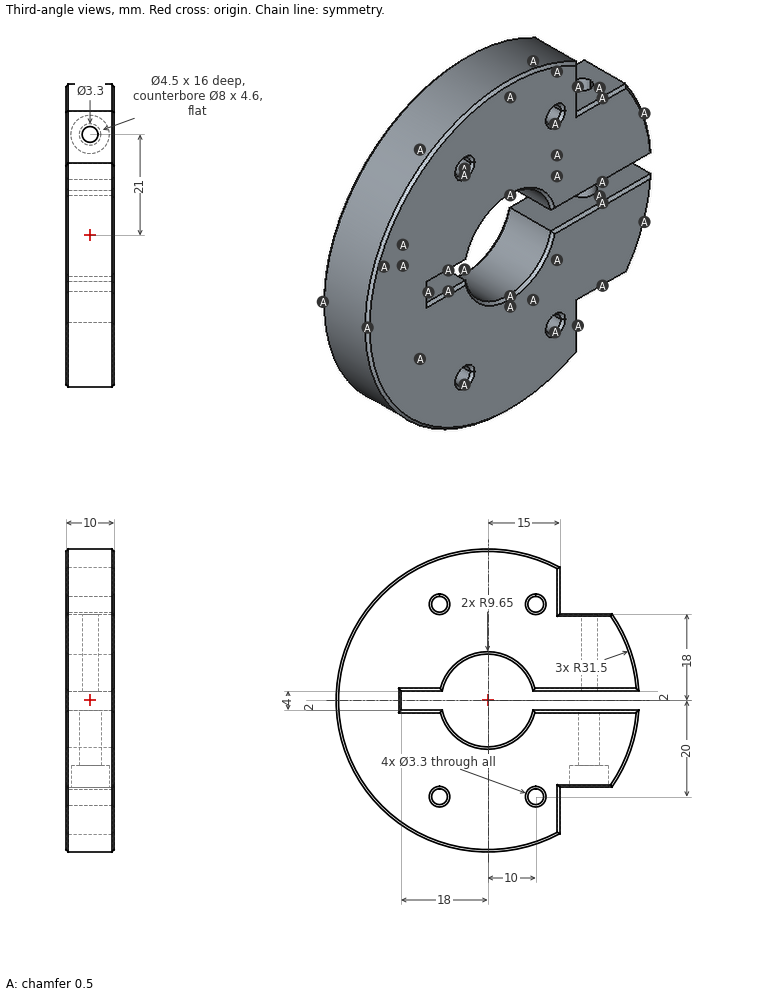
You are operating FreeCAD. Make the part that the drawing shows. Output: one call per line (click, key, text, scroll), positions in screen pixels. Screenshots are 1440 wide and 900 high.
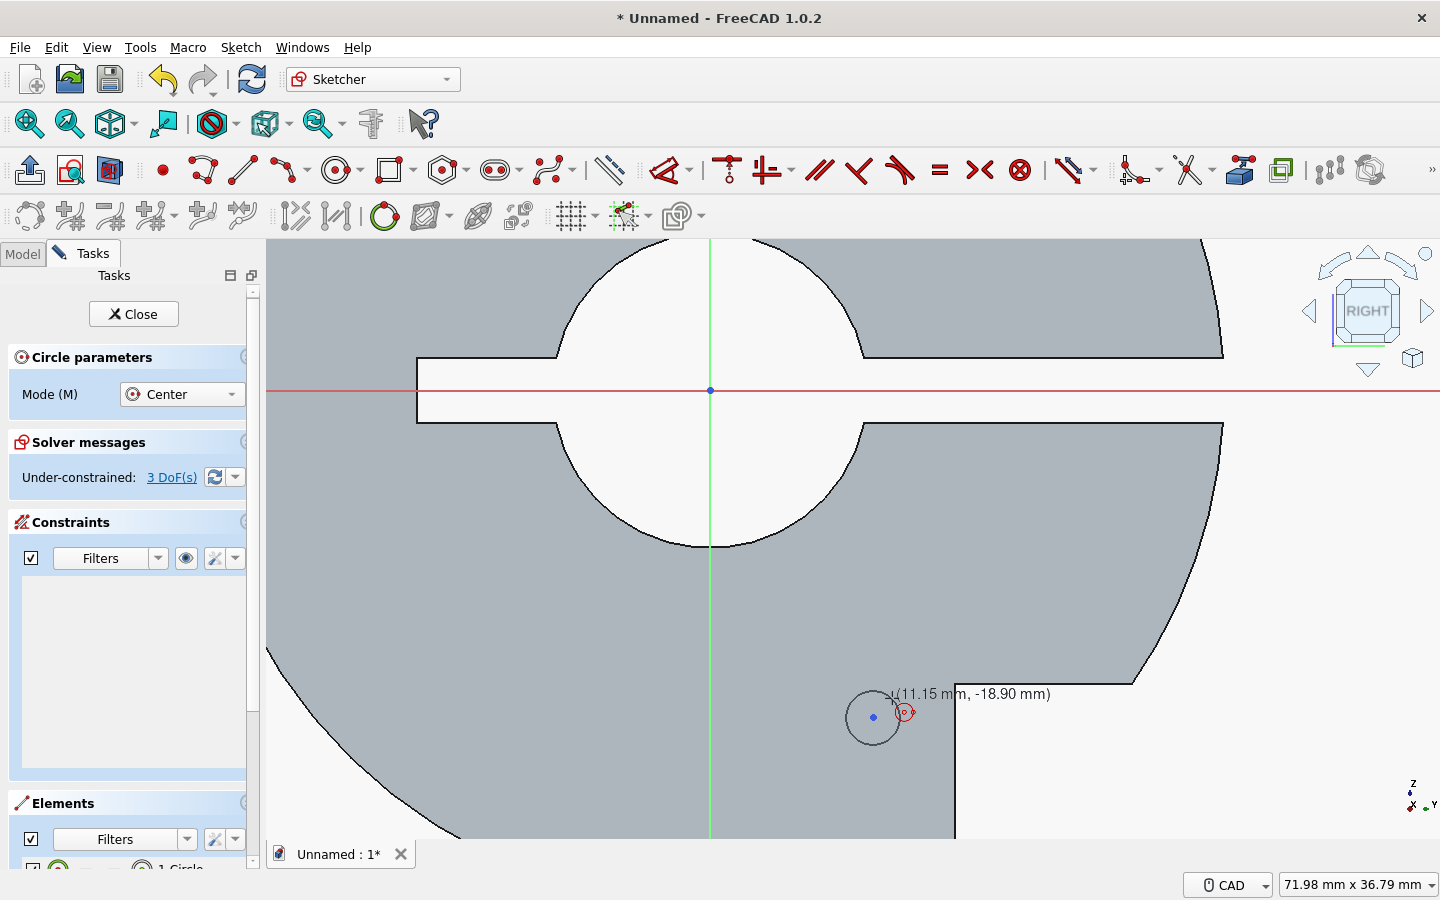
click(547, 717)
click(566, 698)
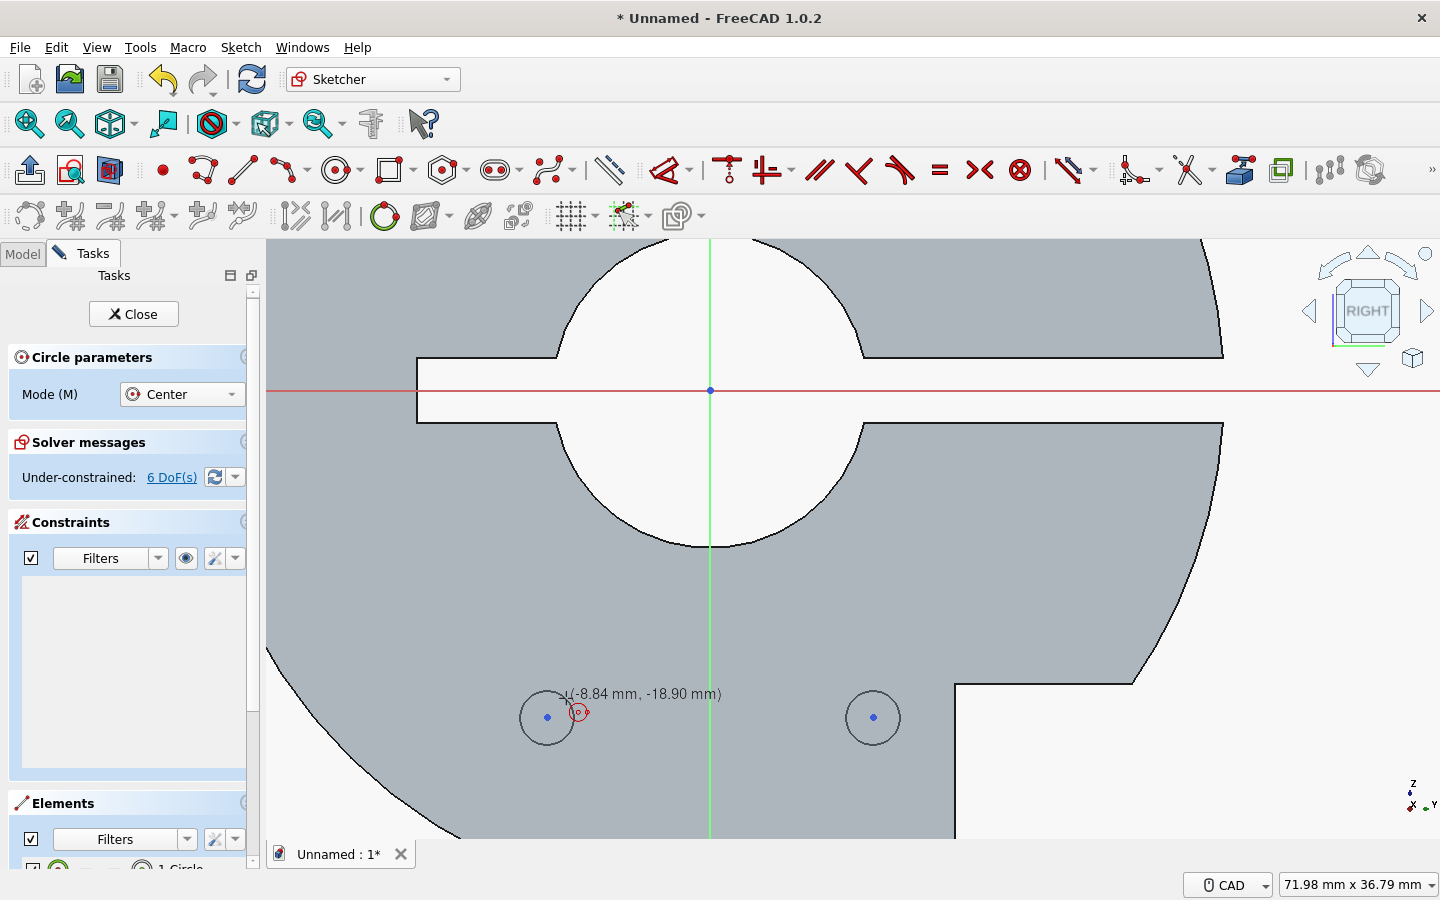
scroll(875, 719, down, 3)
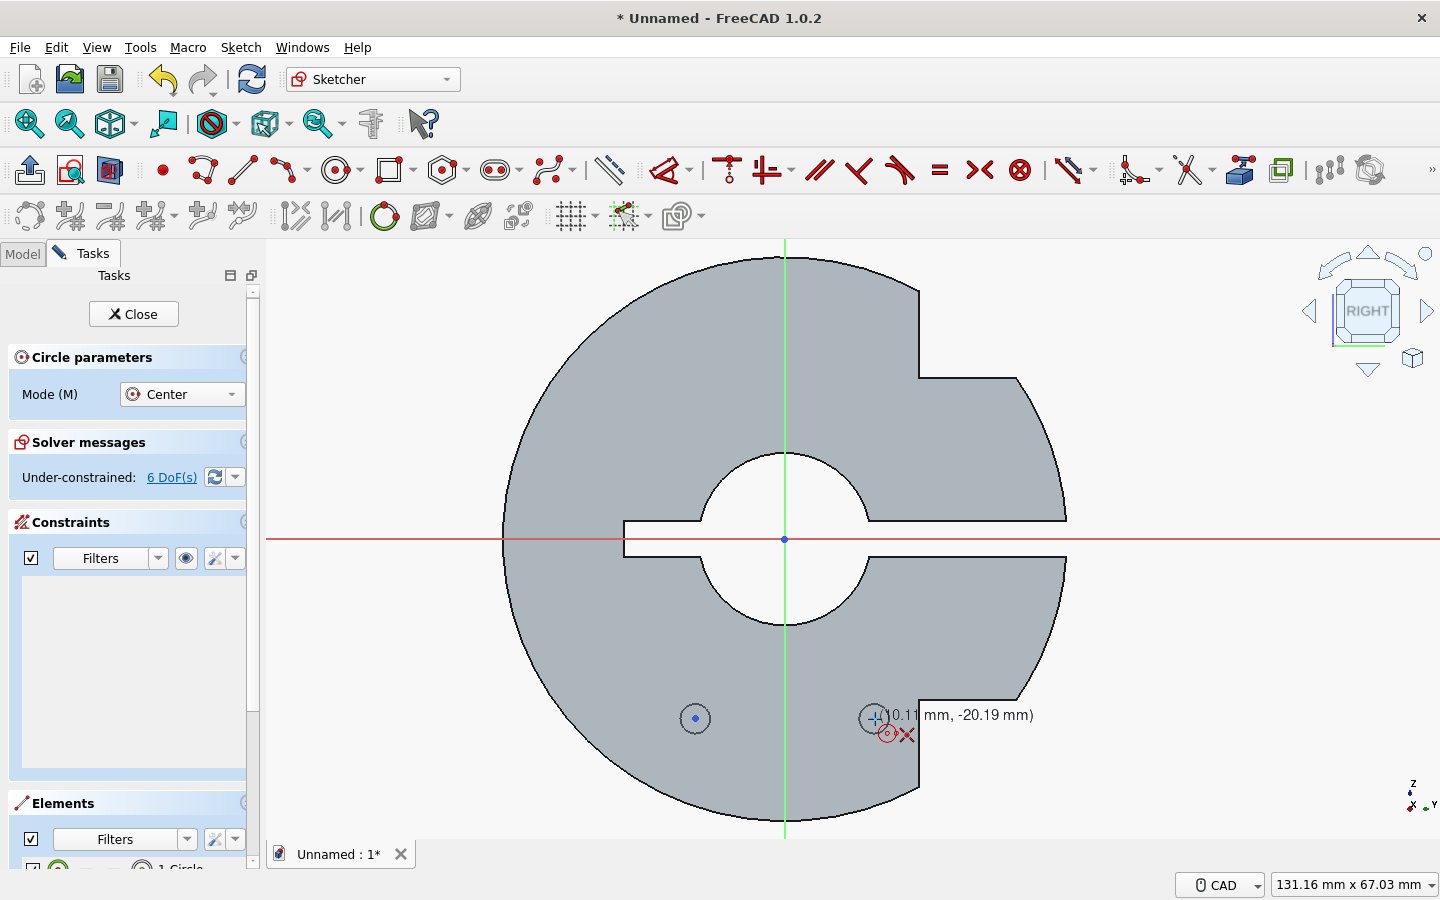
scroll(695, 360, up, 3)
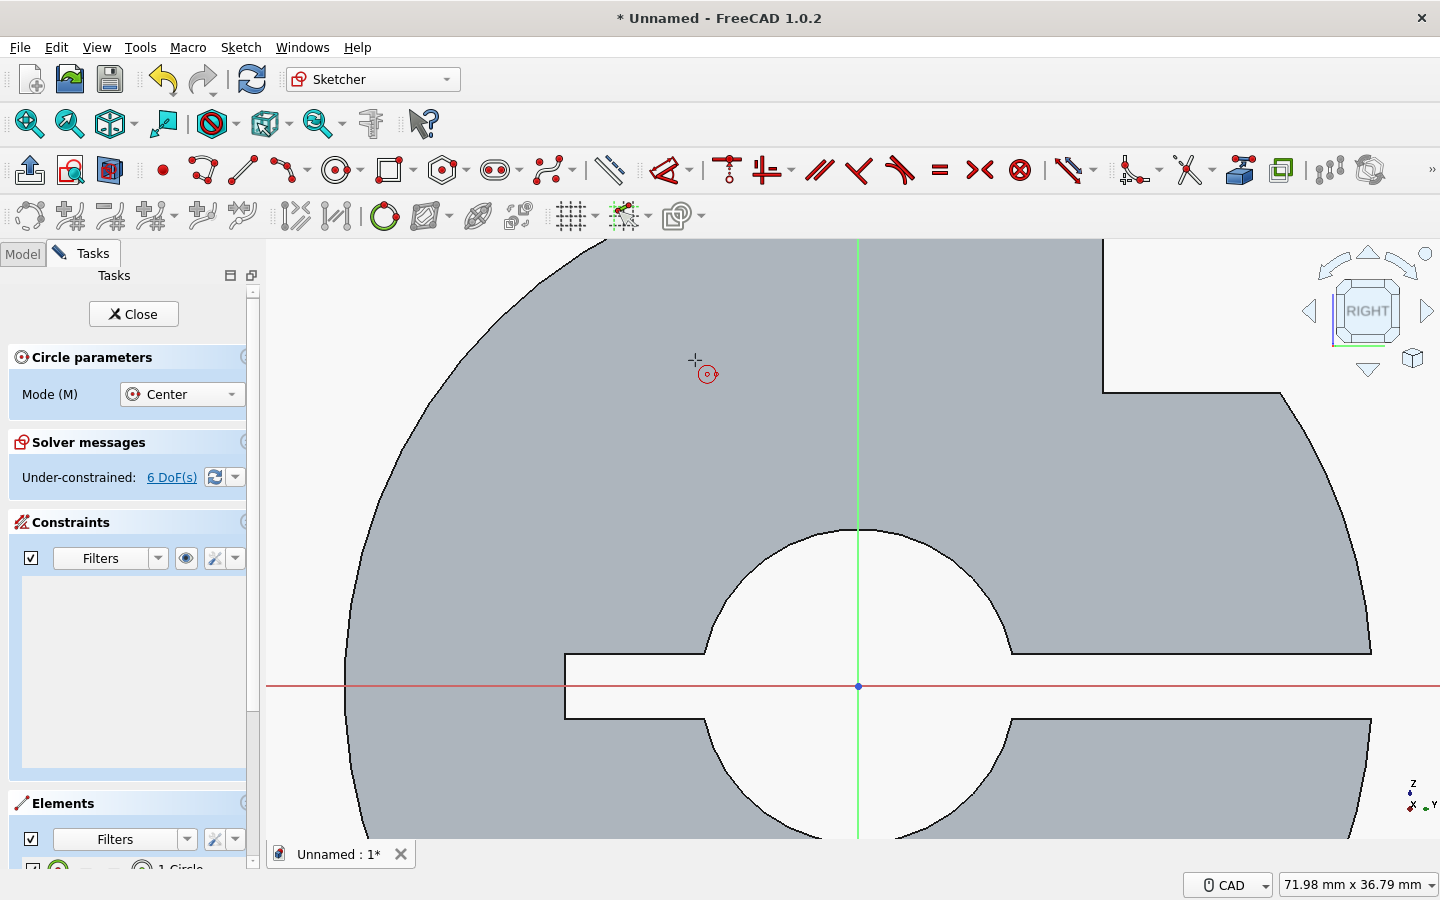
click(695, 360)
click(714, 341)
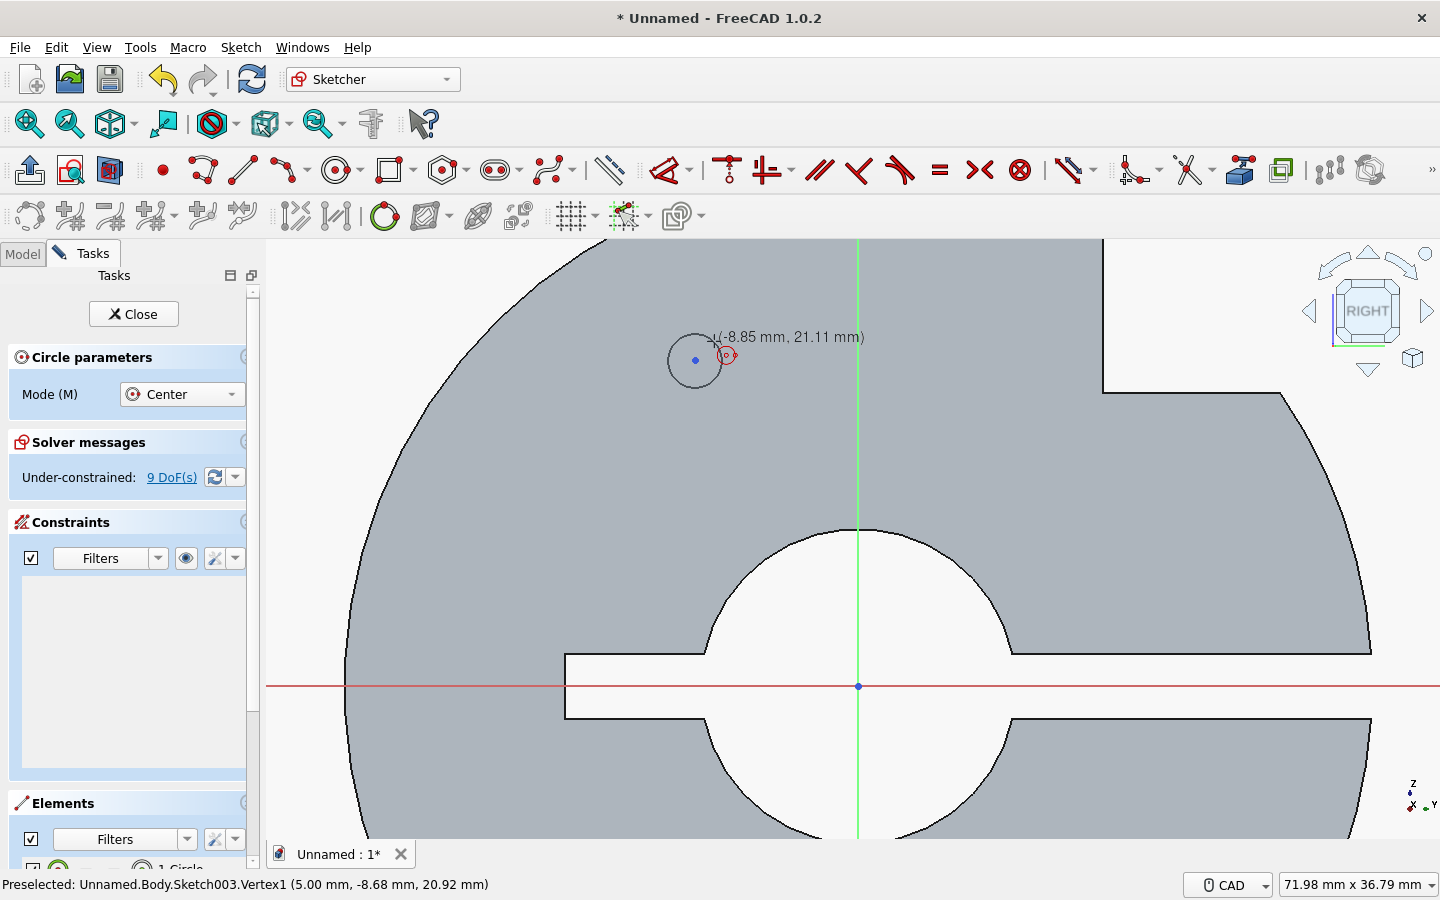
click(1021, 360)
click(1040, 341)
key(Escape)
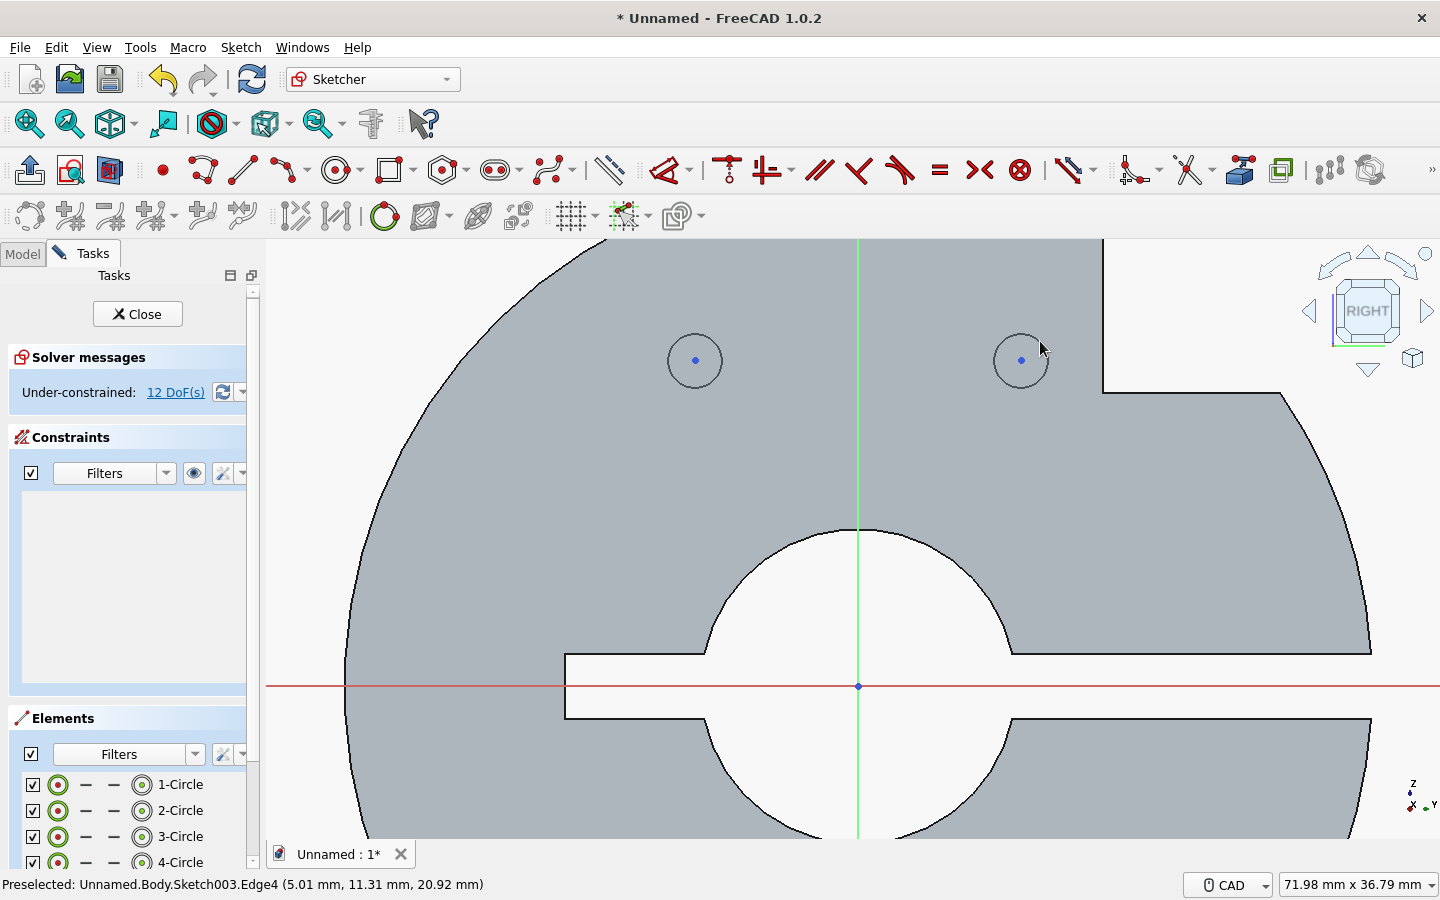
scroll(695, 360, down, 3)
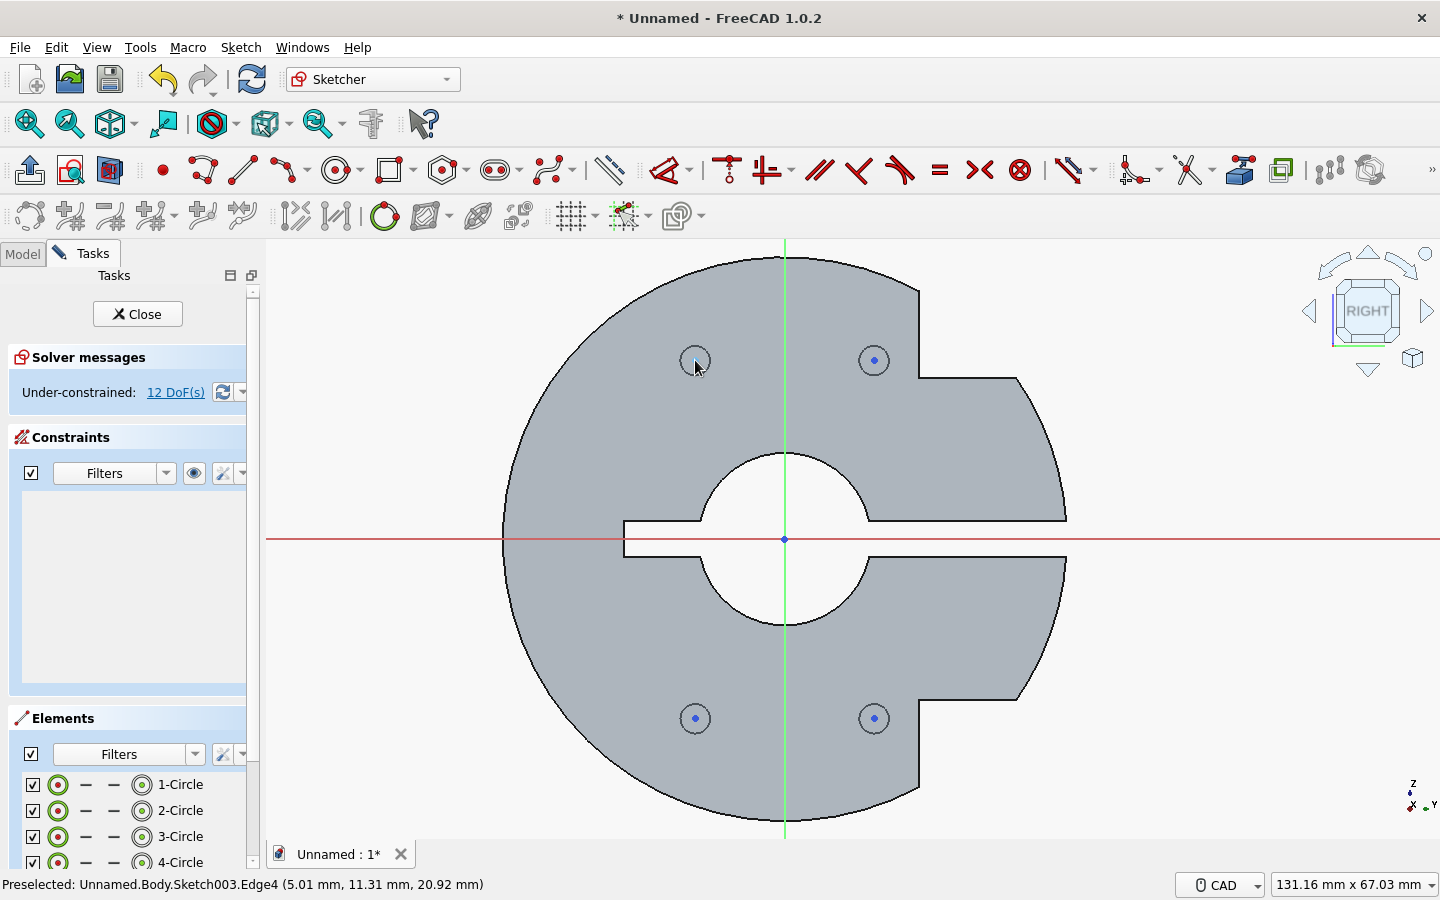
click(885, 708)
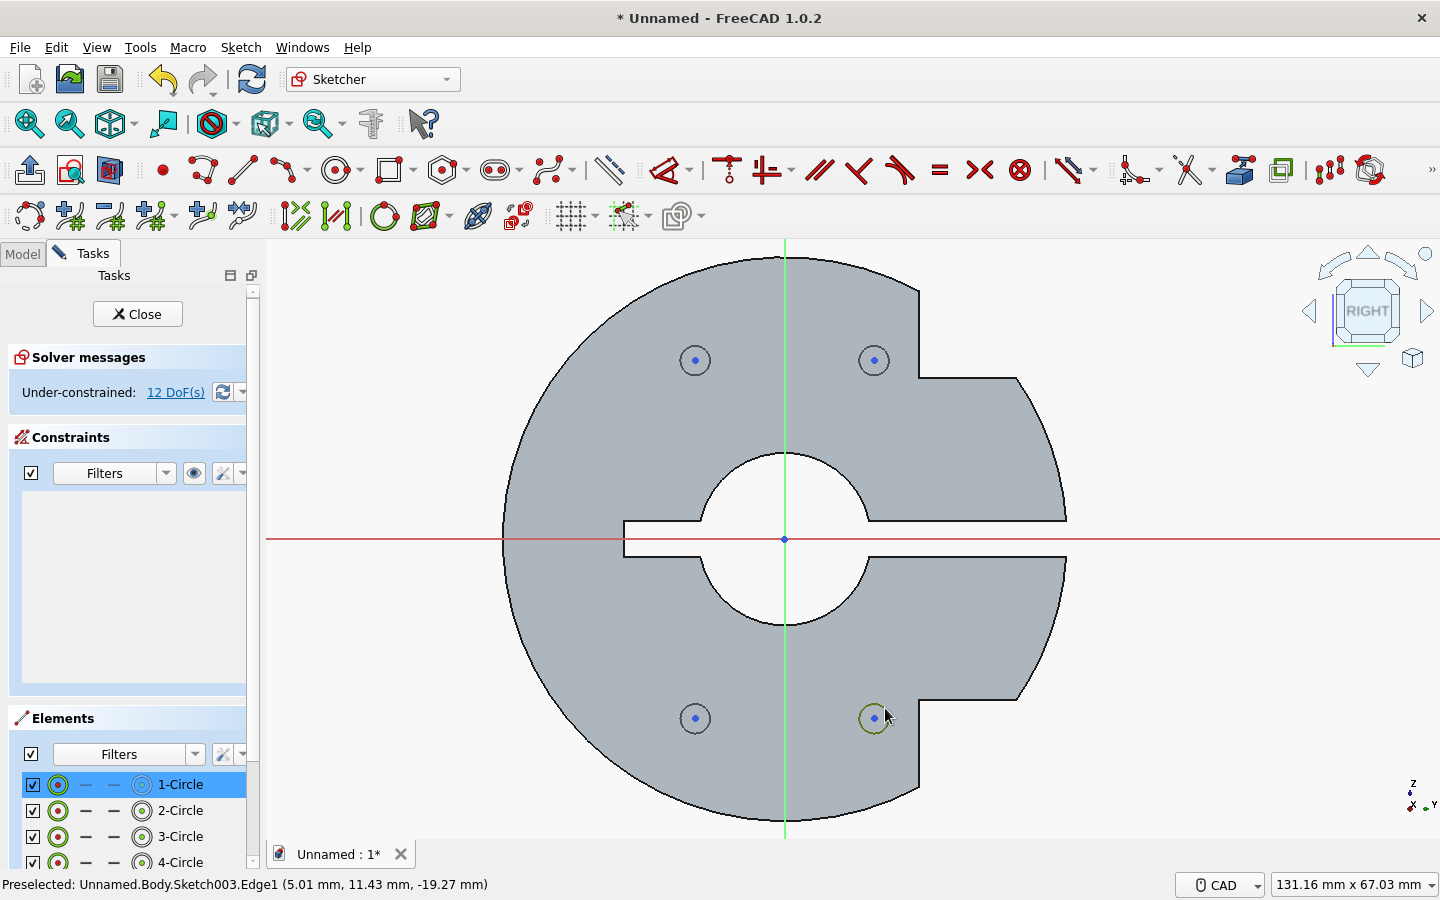
click(706, 708)